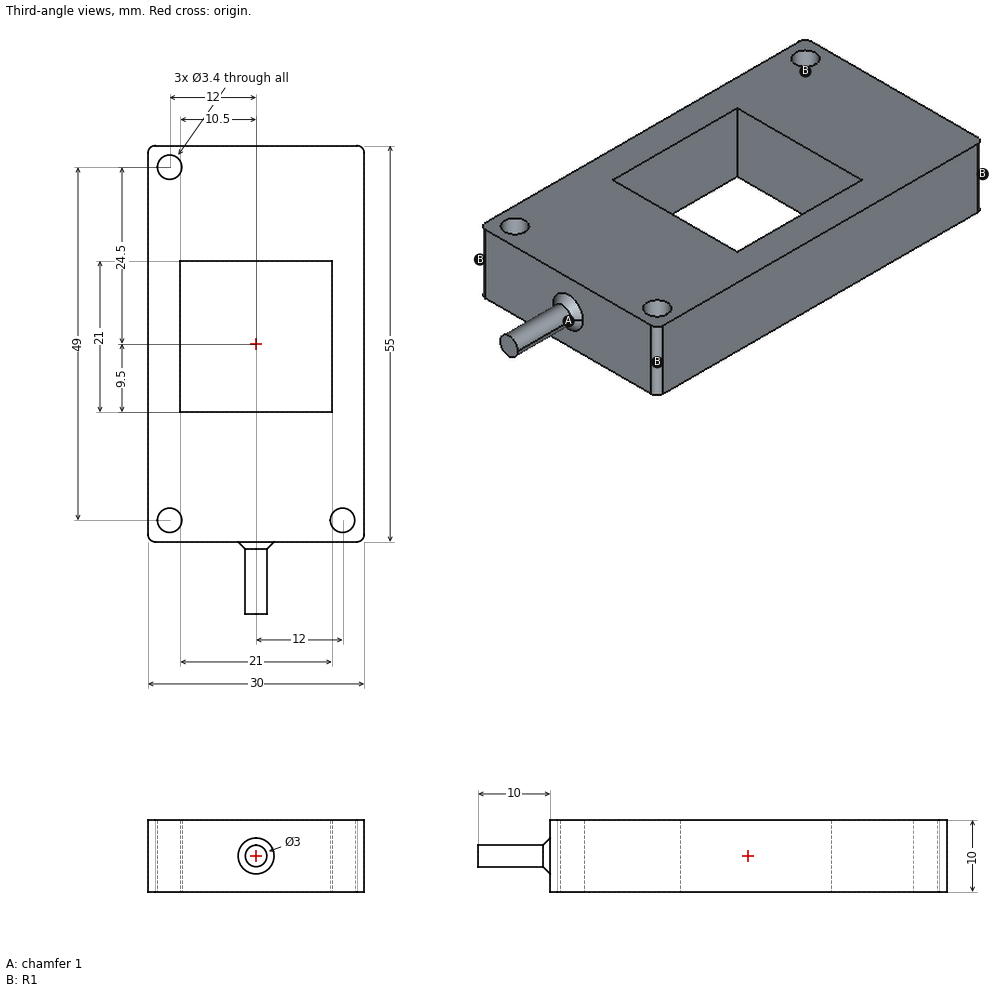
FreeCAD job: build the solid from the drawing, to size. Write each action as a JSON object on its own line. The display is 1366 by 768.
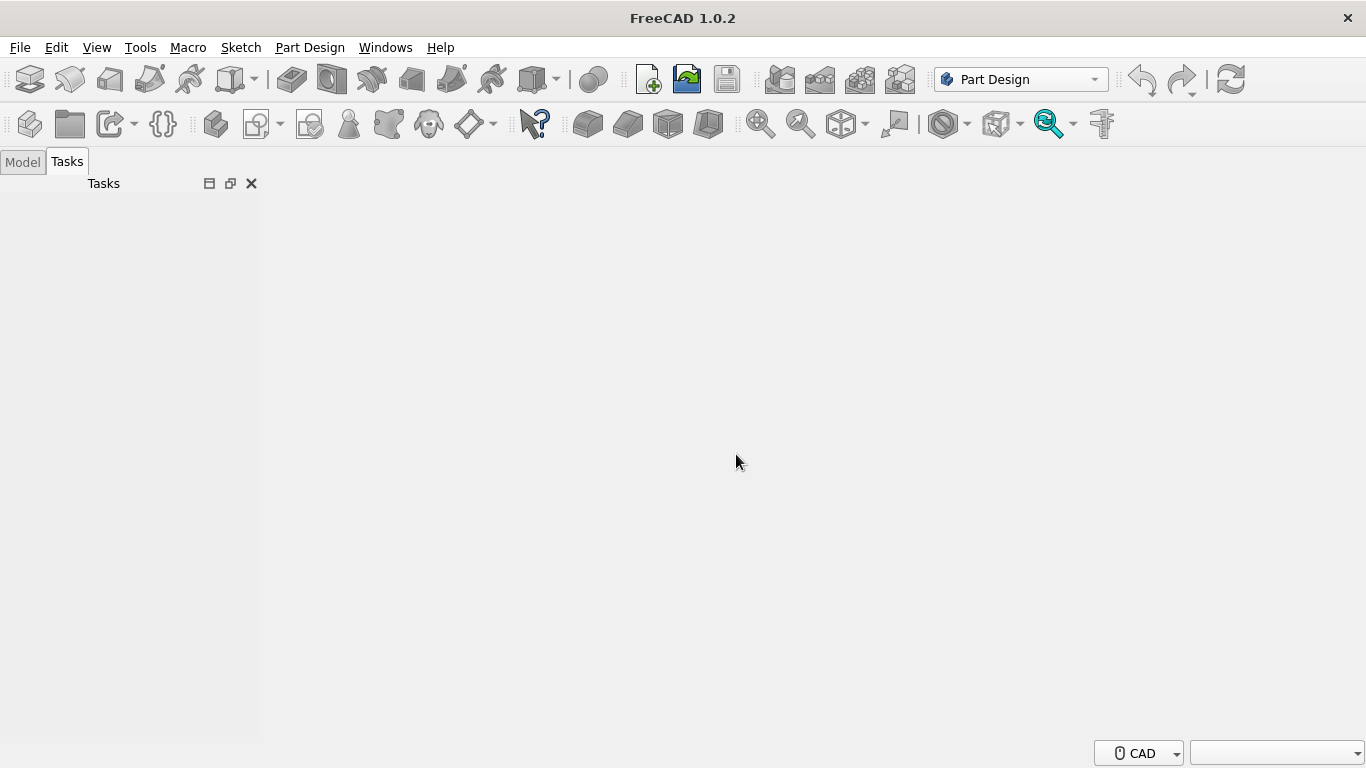
{"action": "left_click", "coordinate": [648, 80]}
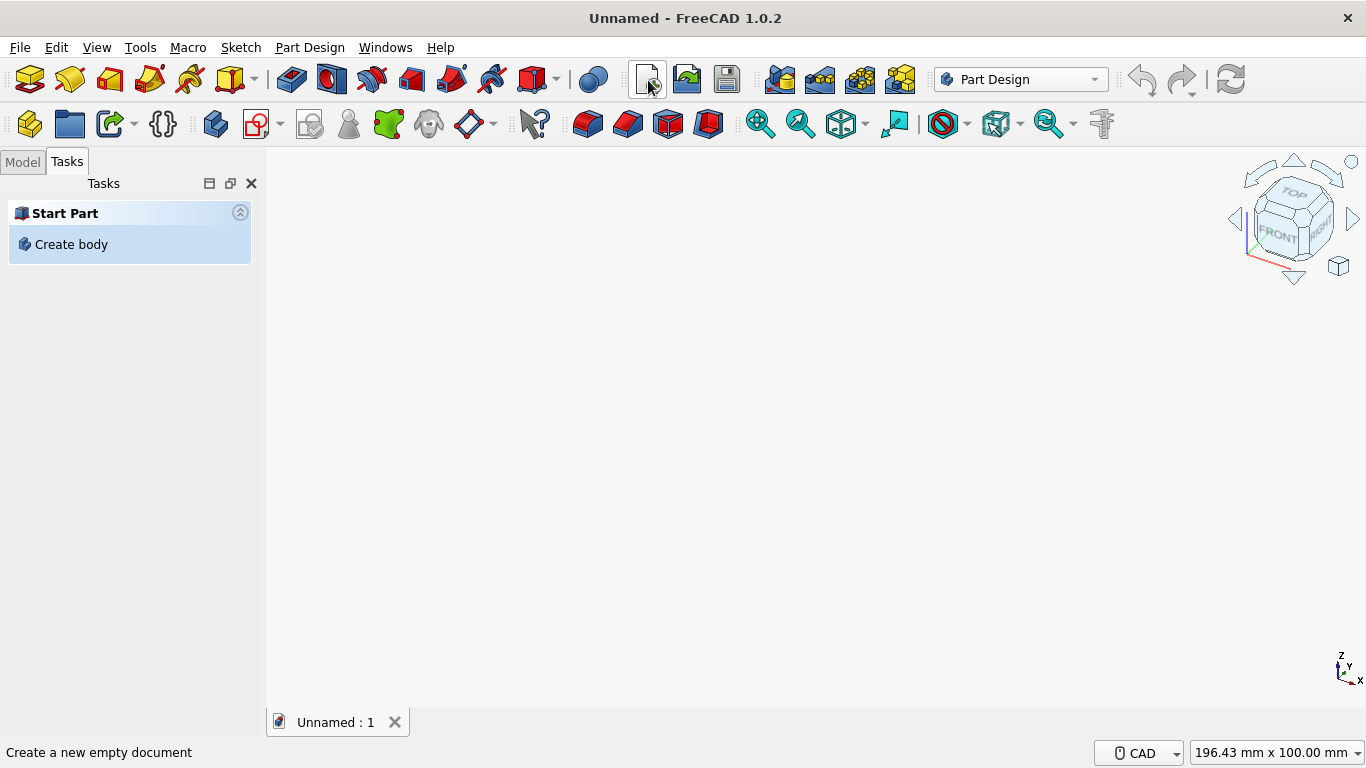
{"action": "left_click", "coordinate": [256, 124]}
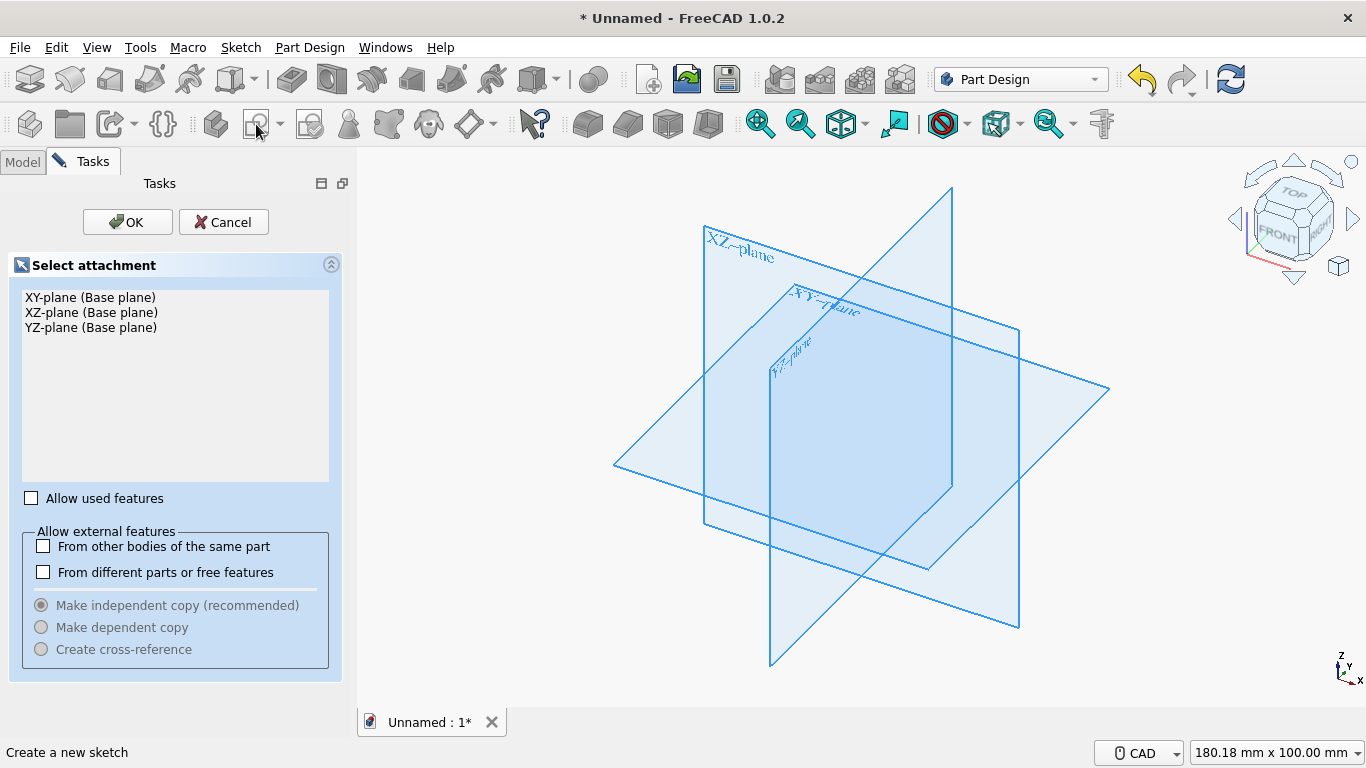
{"action": "left_click", "coordinate": [82, 298]}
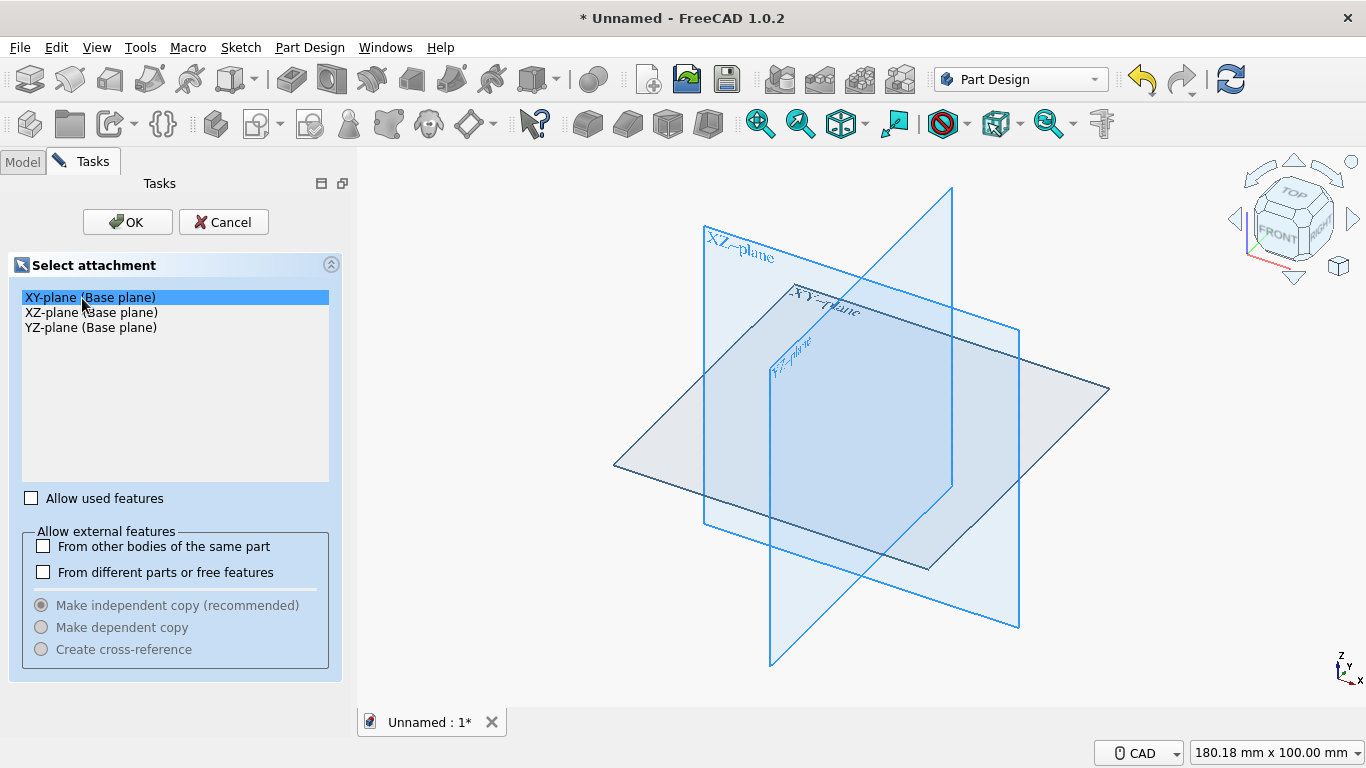
{"action": "left_click", "coordinate": [128, 222]}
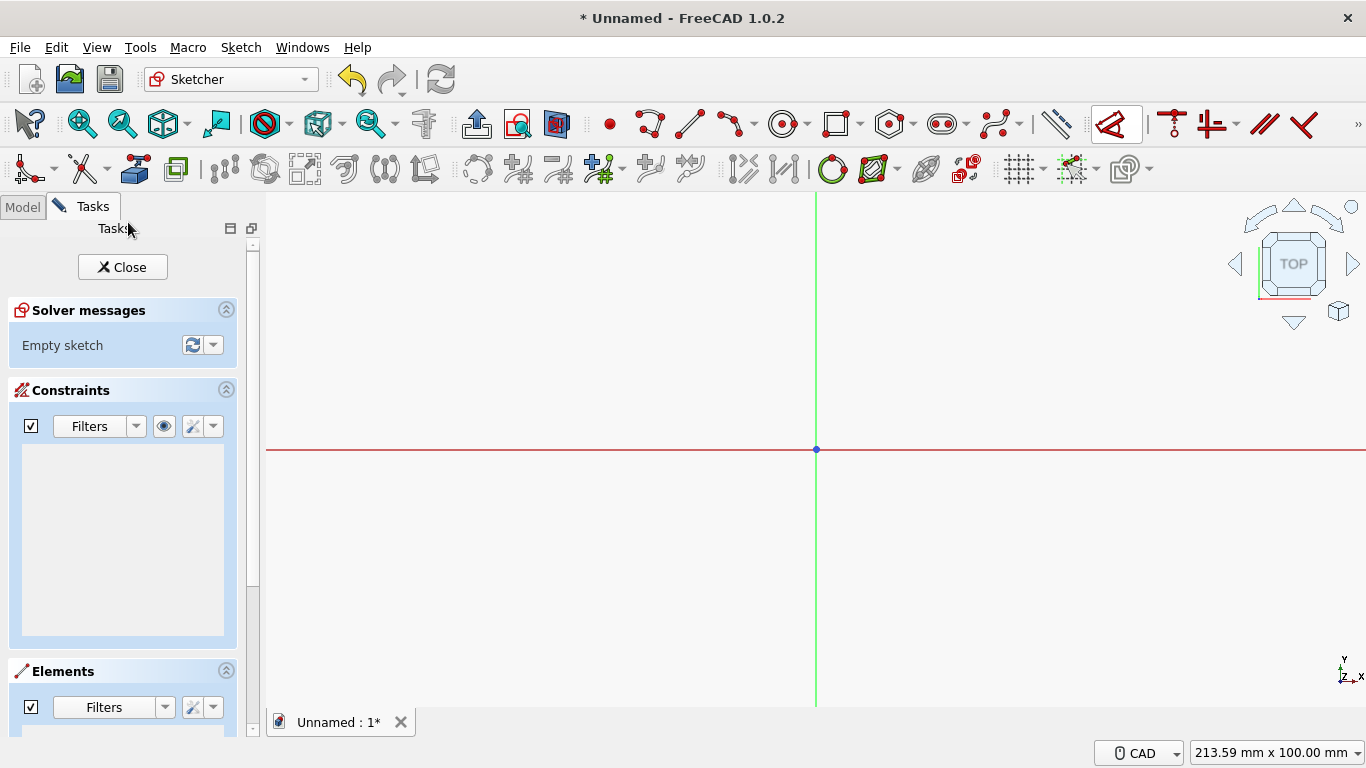
{"action": "key", "text": "g v"}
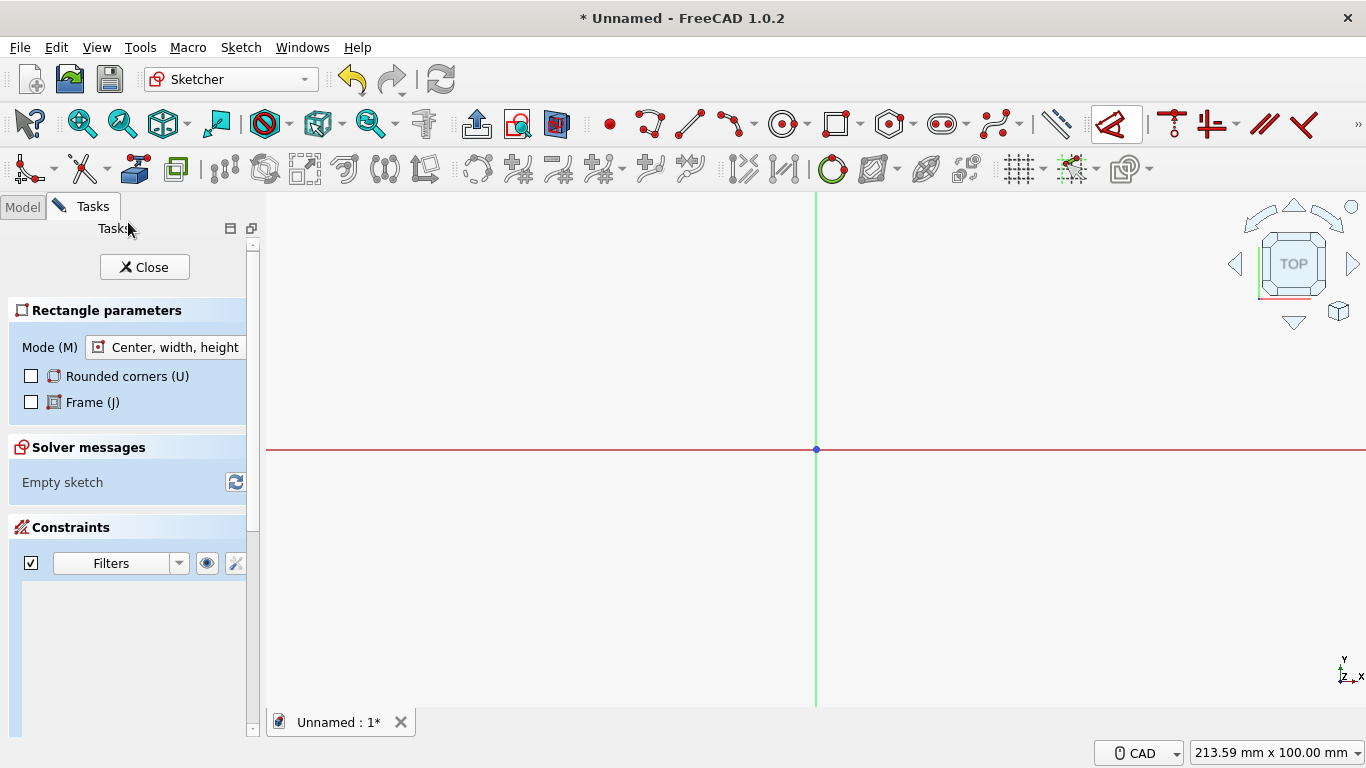
{"action": "left_click", "coordinate": [816, 450]}
{"action": "left_click", "coordinate": [893, 308]}
{"action": "key", "text": "Escape"}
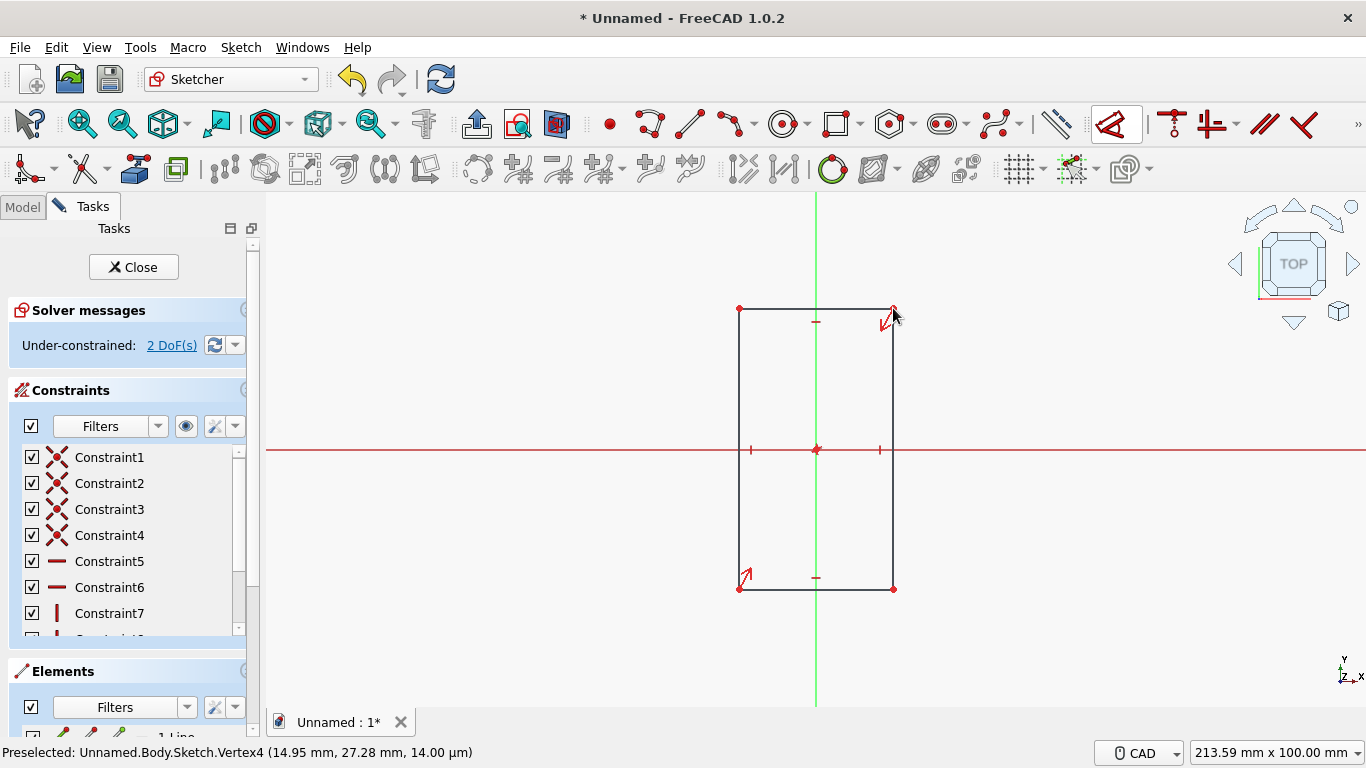
{"action": "key", "text": "d"}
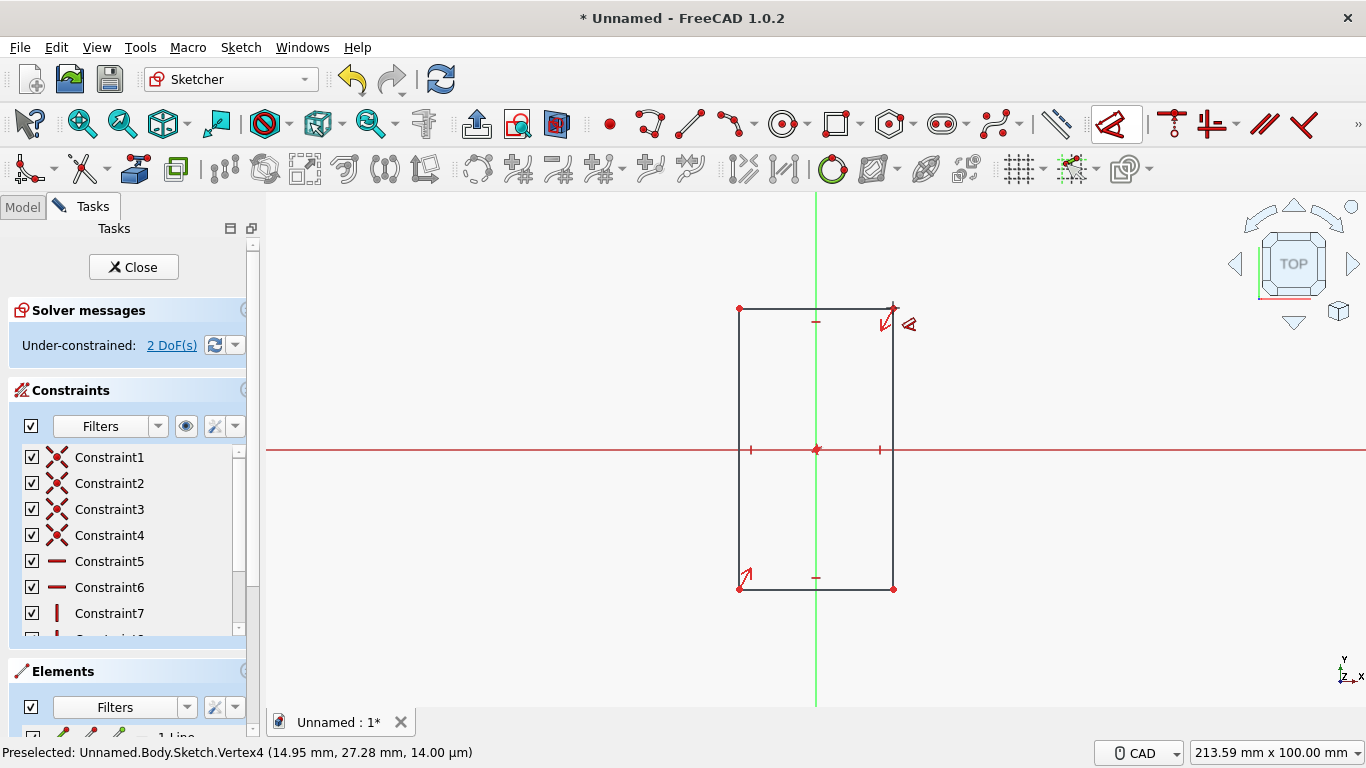
{"action": "left_click", "coordinate": [785, 590]}
{"action": "left_click", "coordinate": [781, 624]}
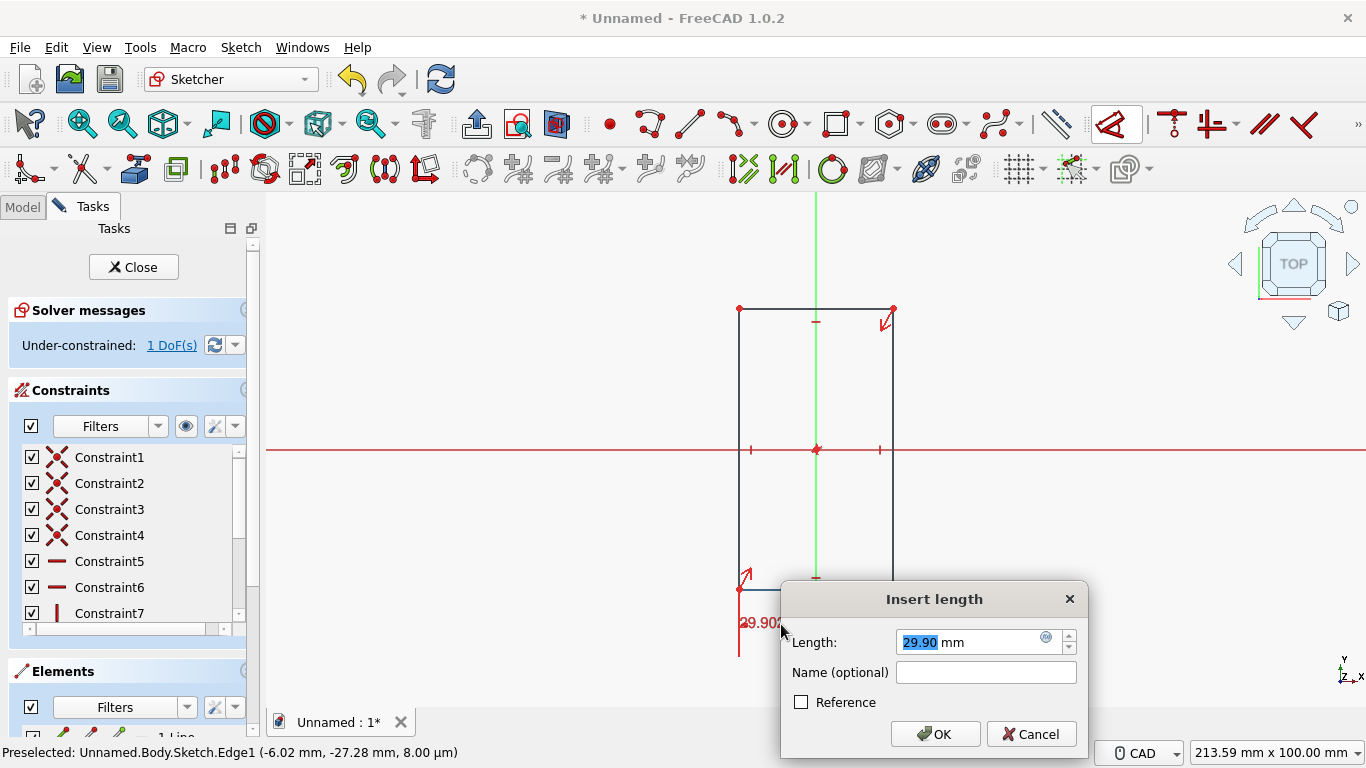
{"action": "type", "text": "30"}
{"action": "key", "text": "Return"}